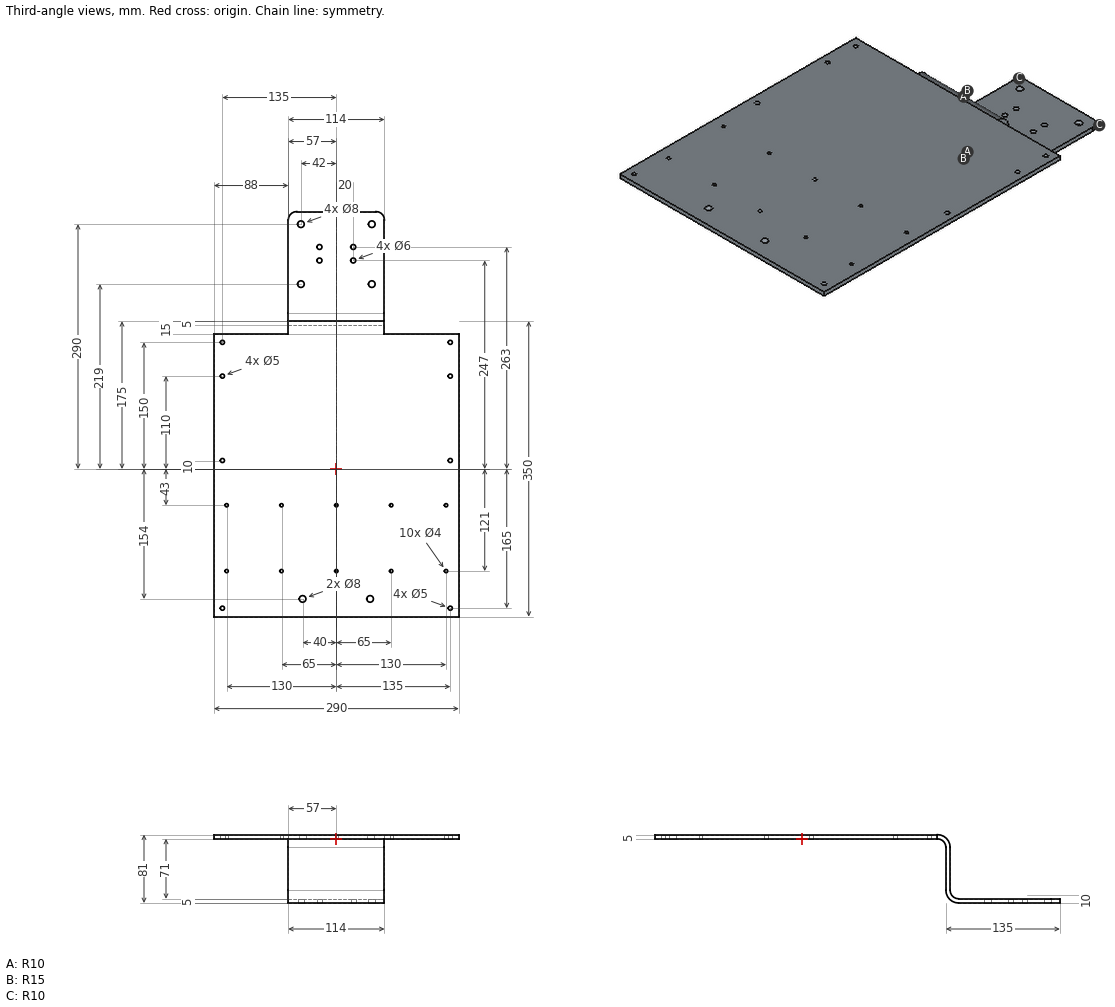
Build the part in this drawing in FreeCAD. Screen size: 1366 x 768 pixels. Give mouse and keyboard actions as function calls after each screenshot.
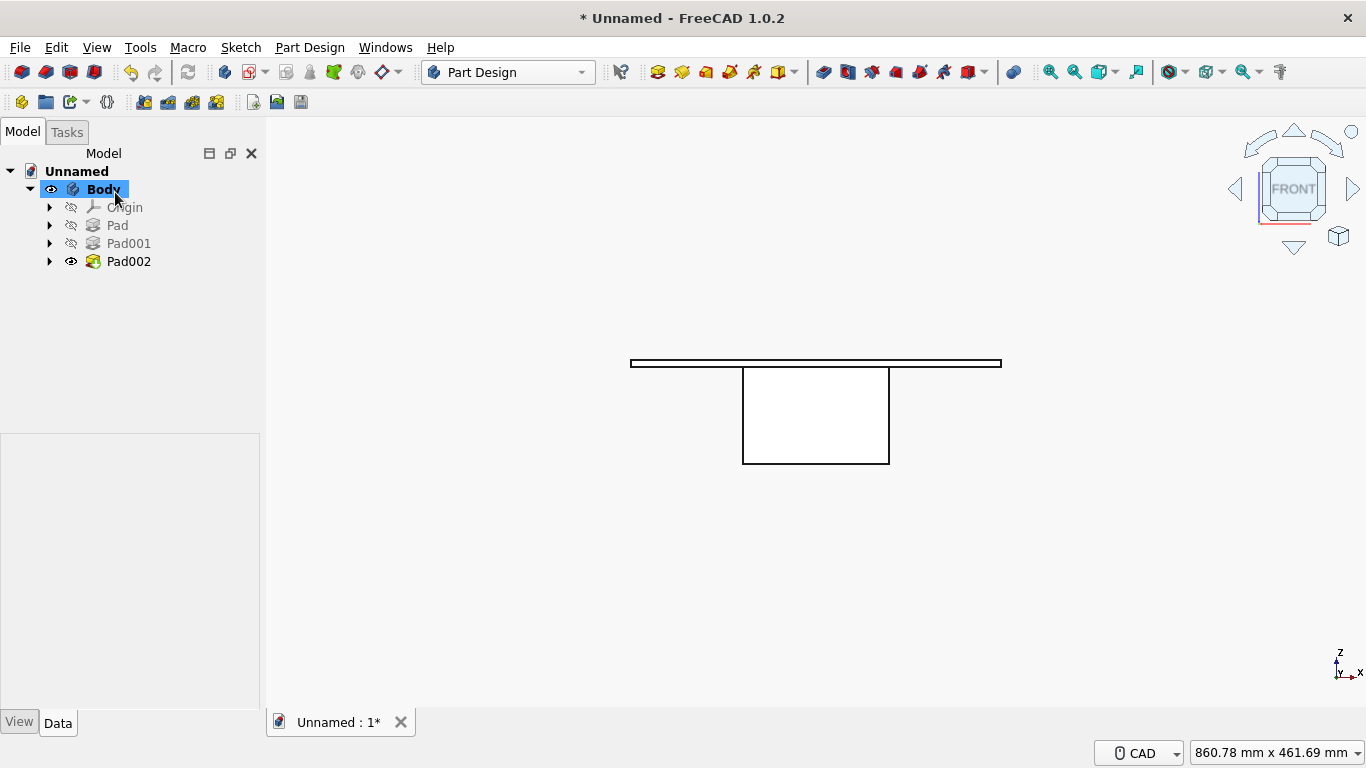
click(1052, 72)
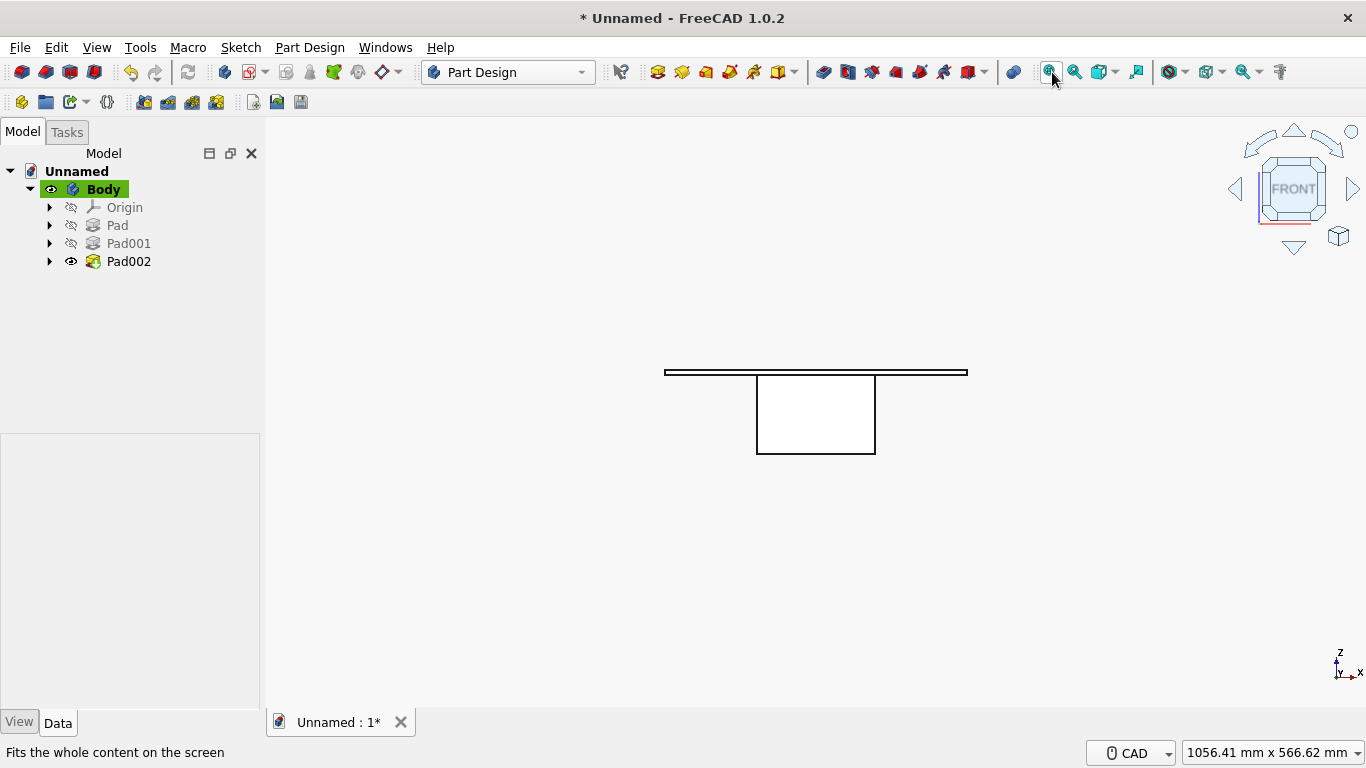
key(0)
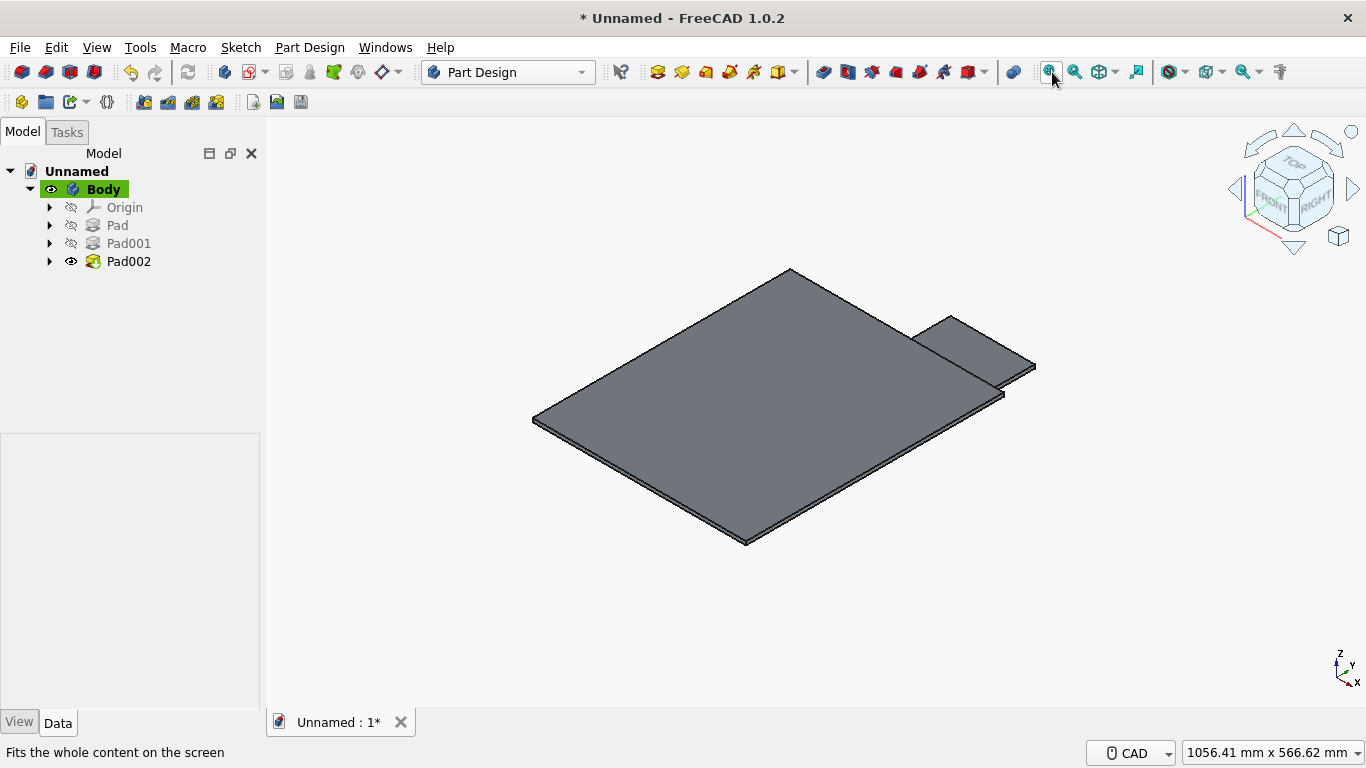
key(2)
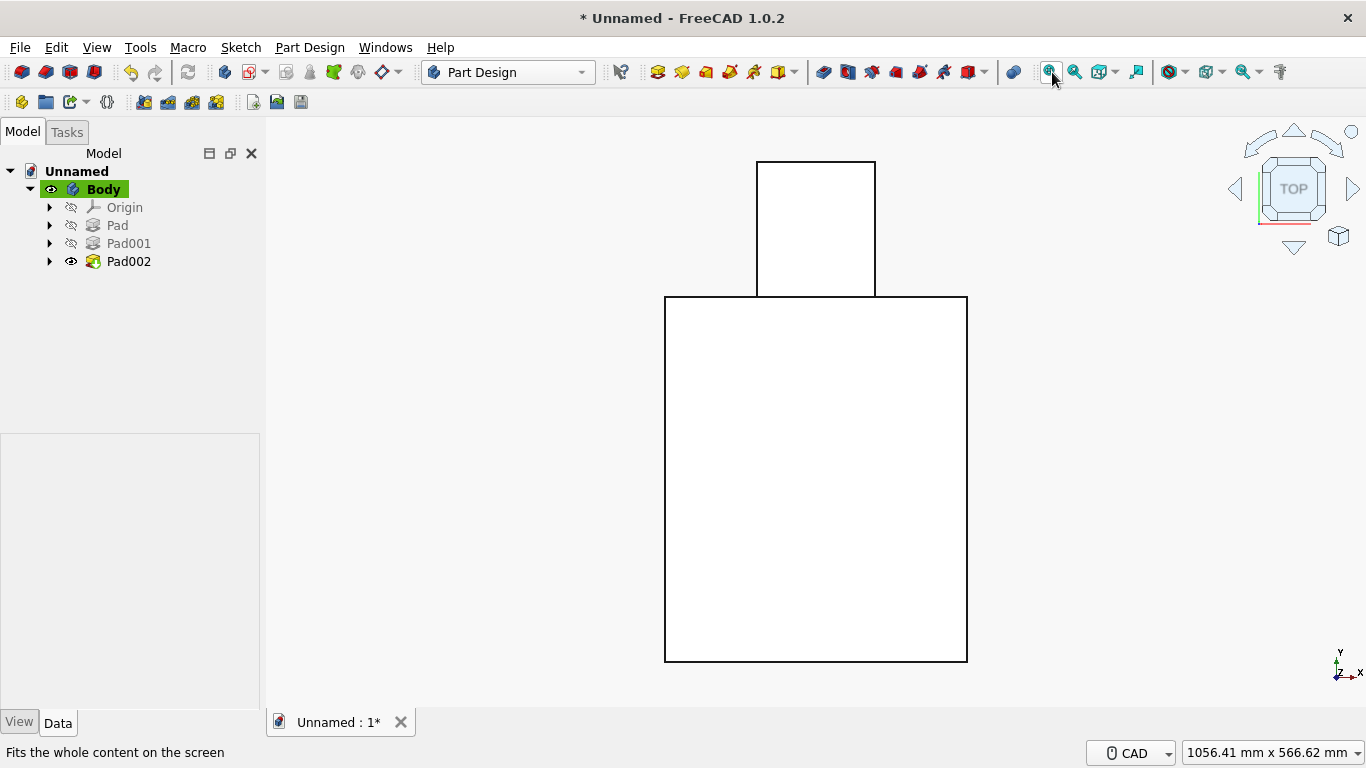
key(1)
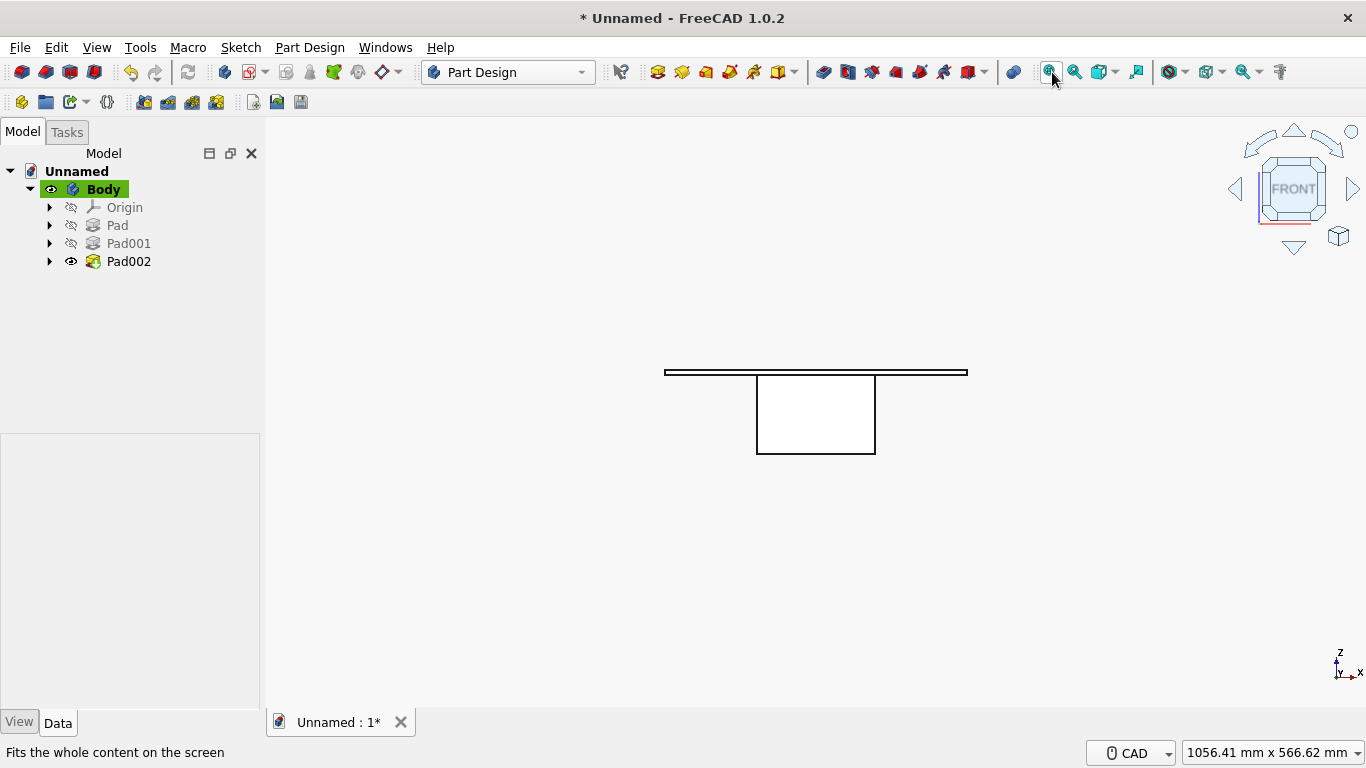
click(1052, 72)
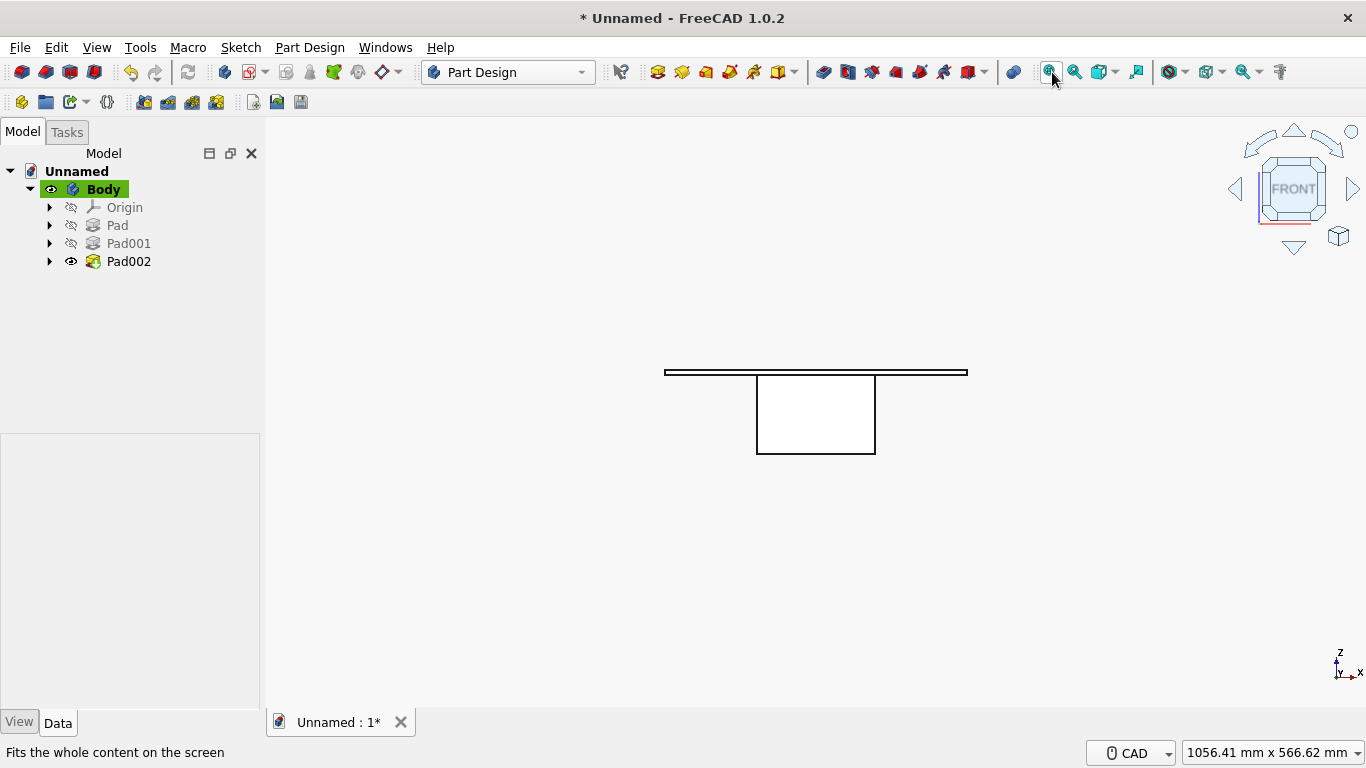
key(3)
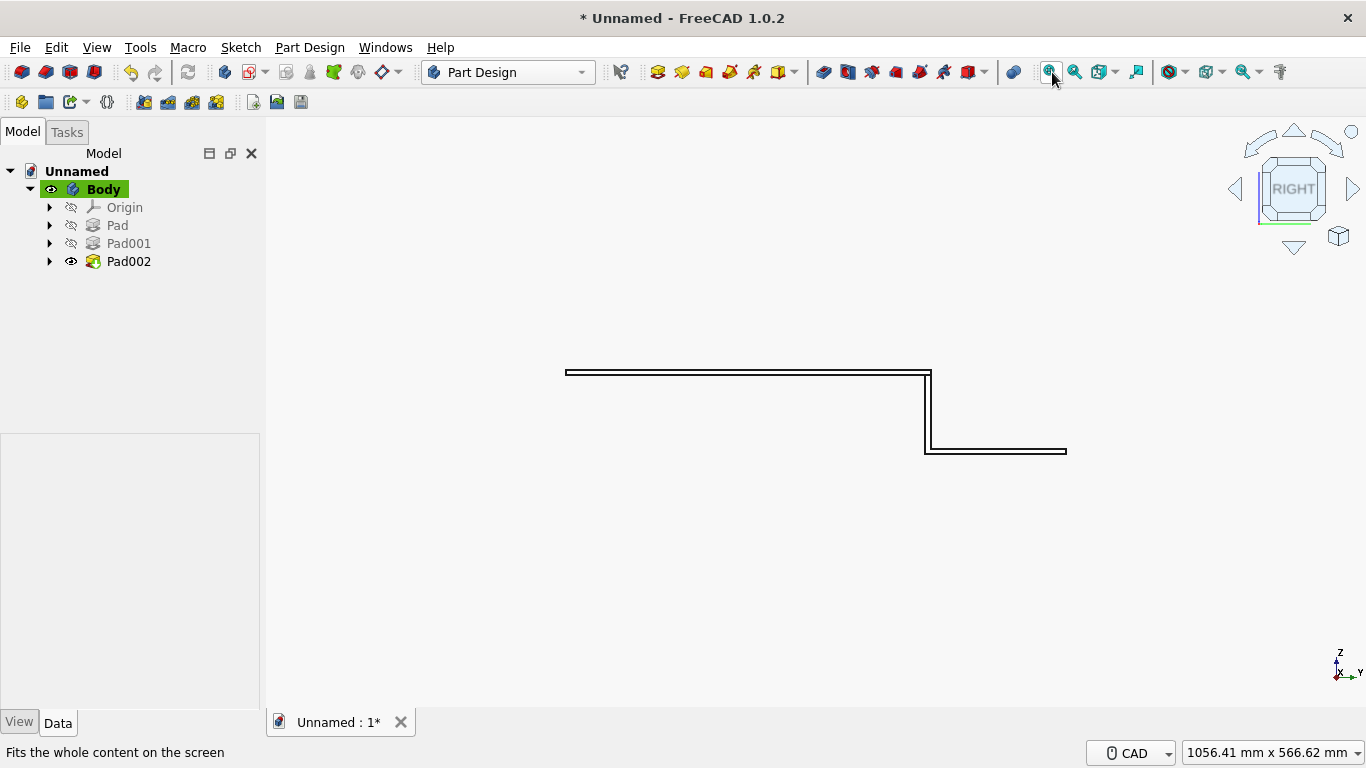
key(5)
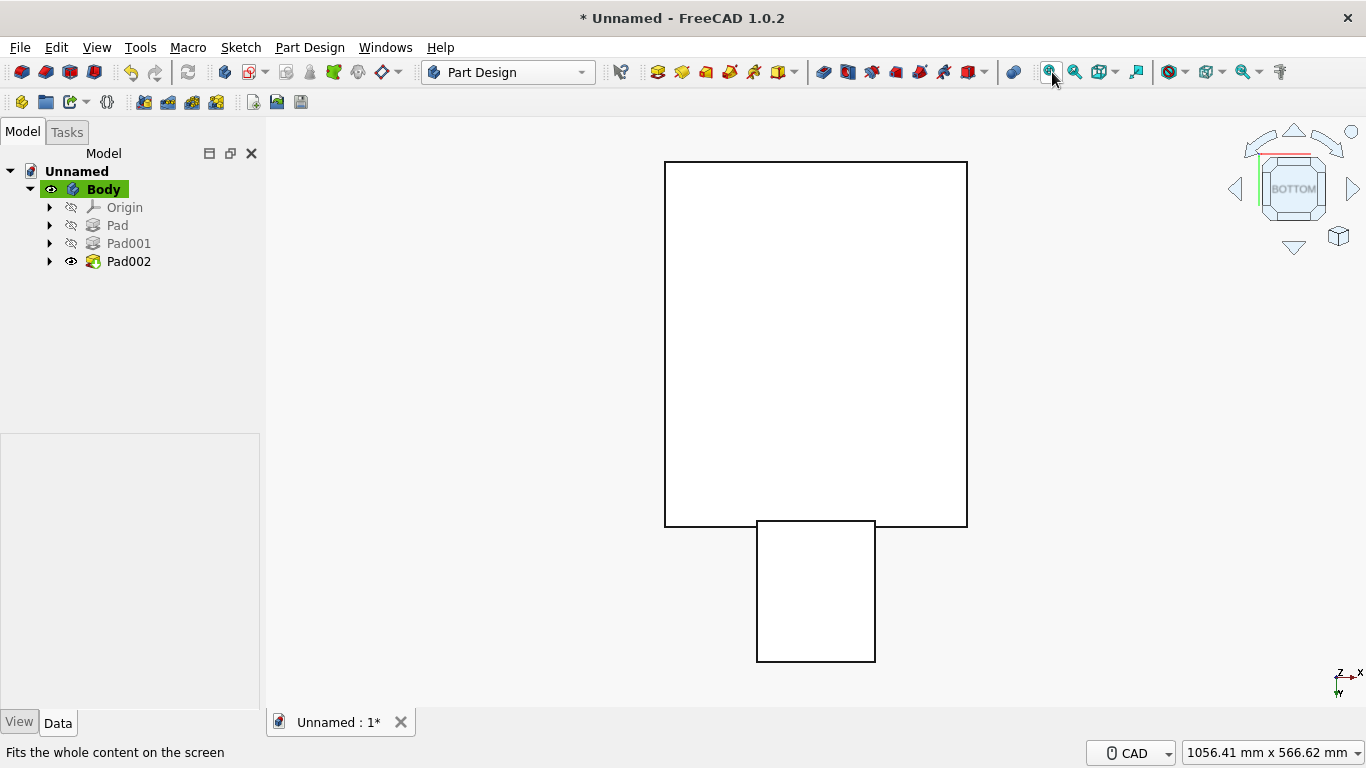
key(4)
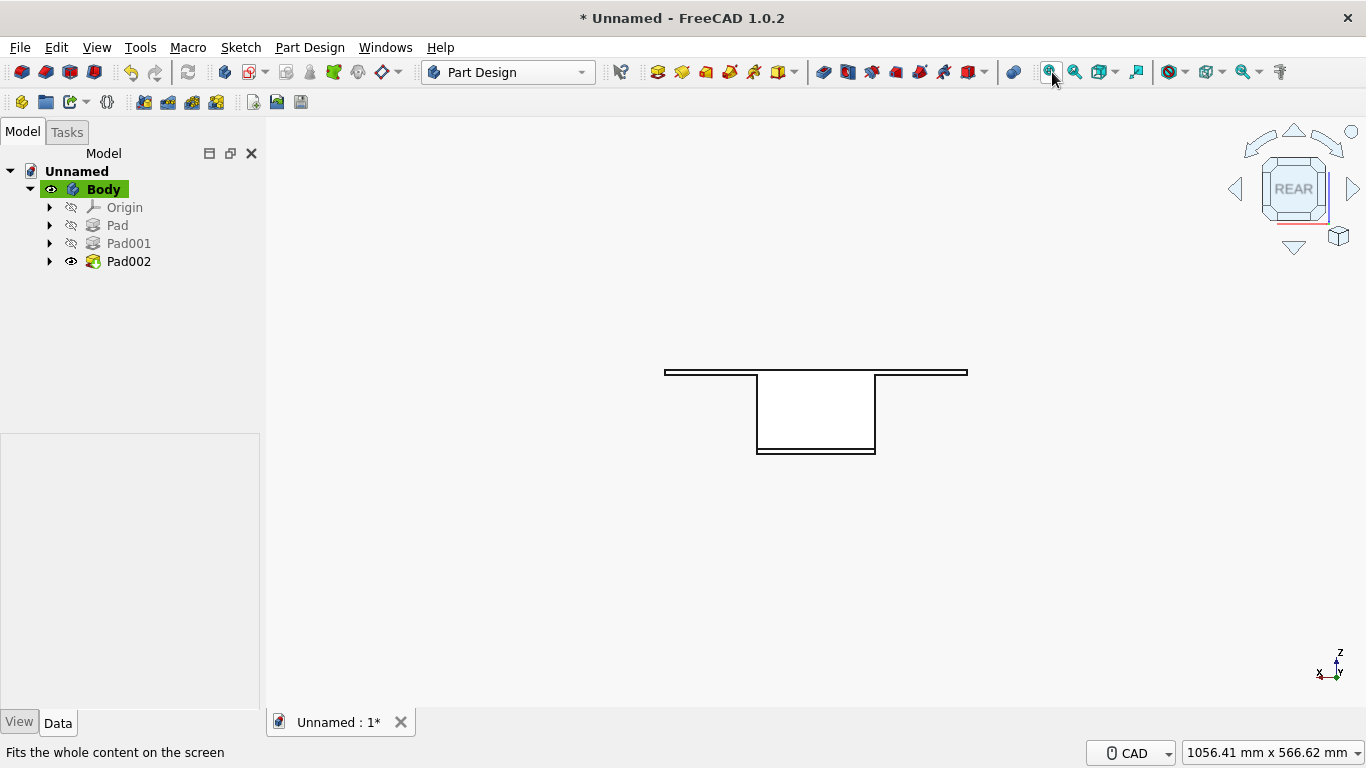
click(1052, 72)